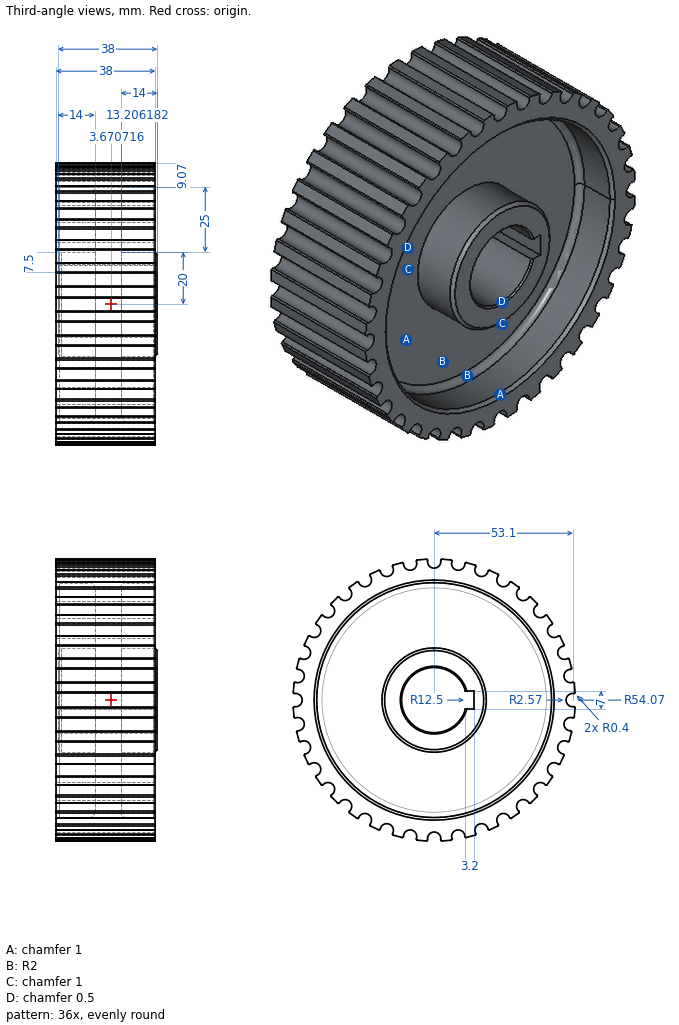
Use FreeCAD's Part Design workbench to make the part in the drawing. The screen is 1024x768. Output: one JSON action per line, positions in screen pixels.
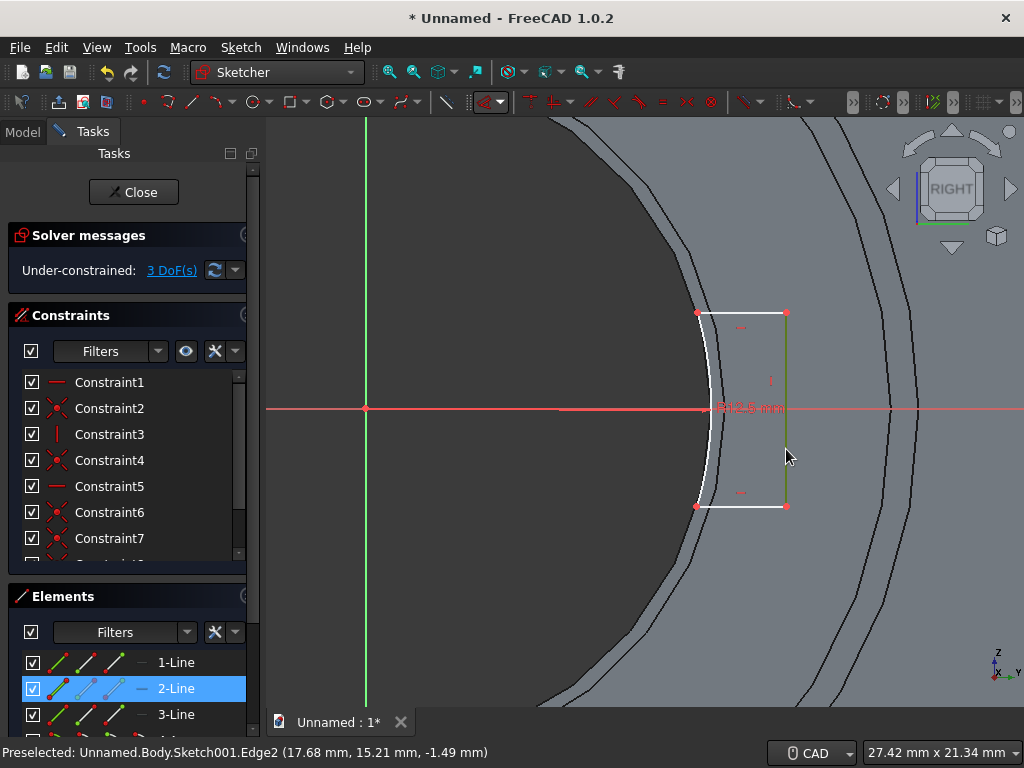
{"action": "key", "text": "i"}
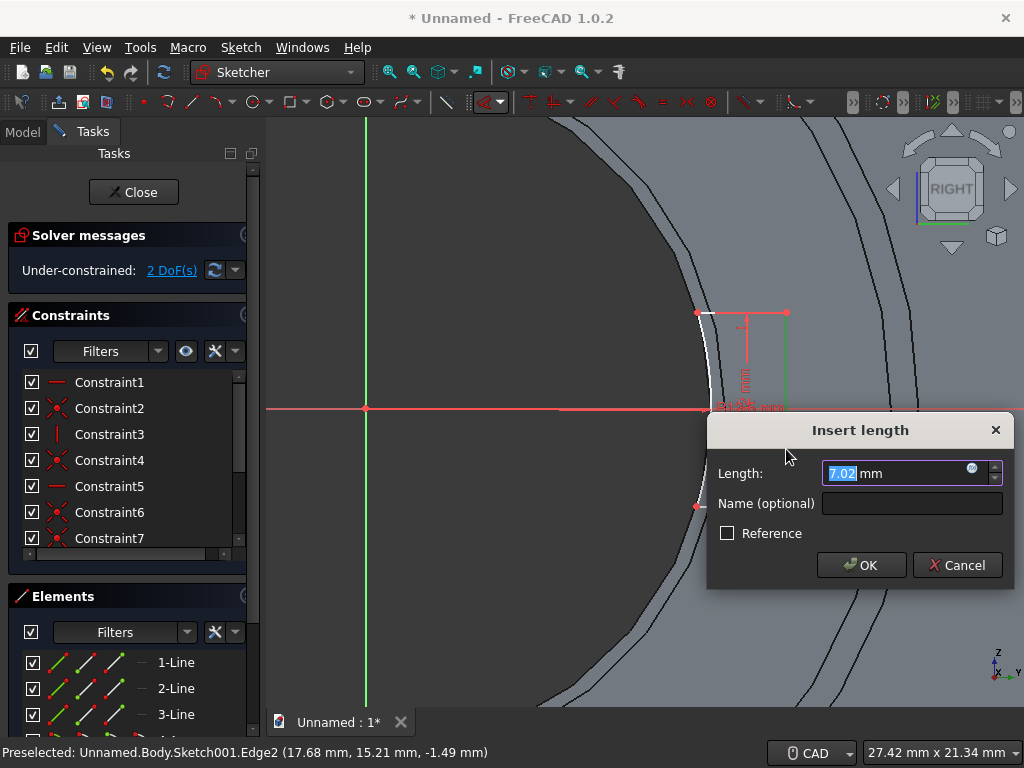
{"action": "type", "text": "7"}
{"action": "key", "text": "Return"}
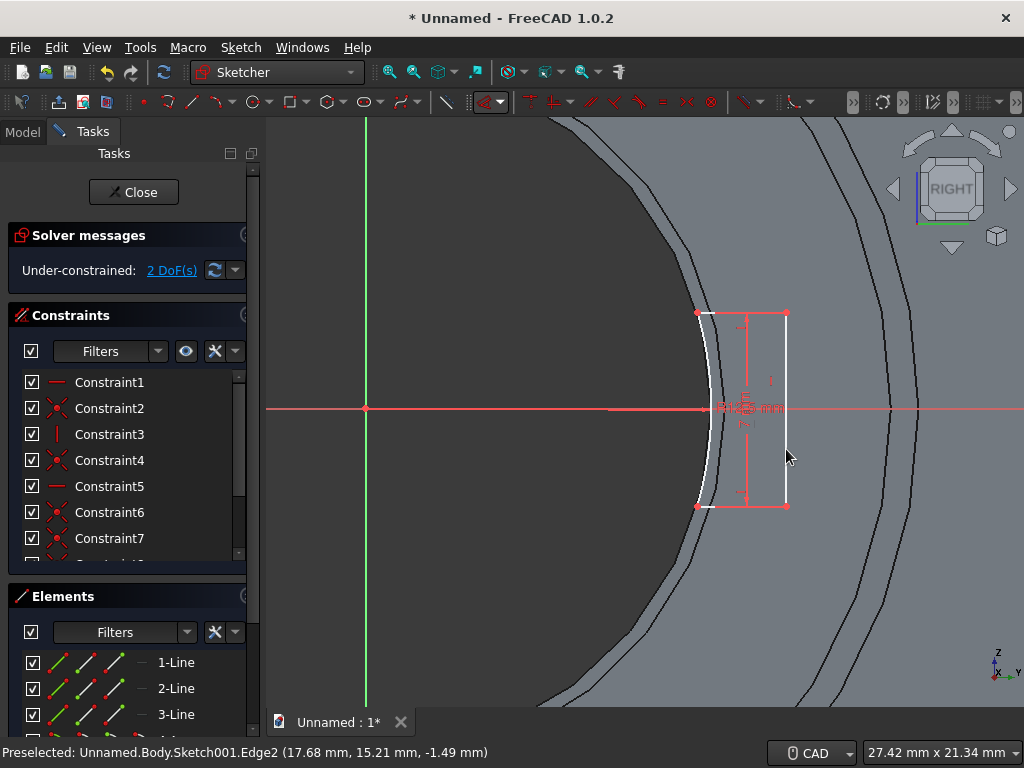
{"action": "left_click", "coordinate": [724, 507]}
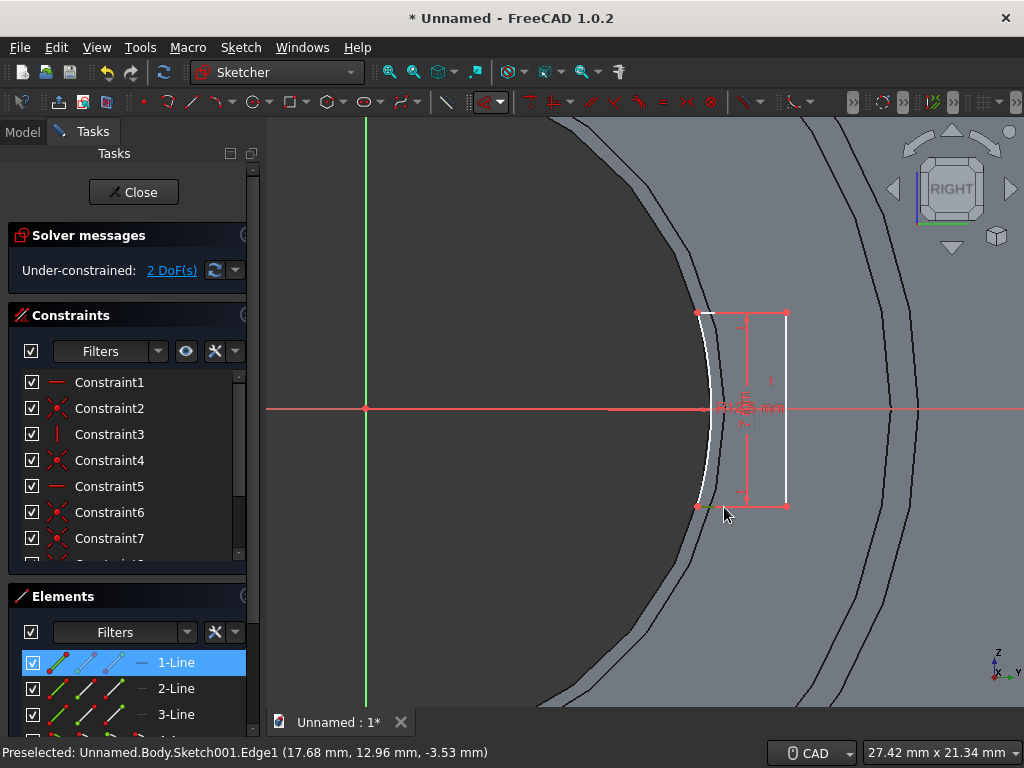
{"action": "left_click", "coordinate": [502, 102]}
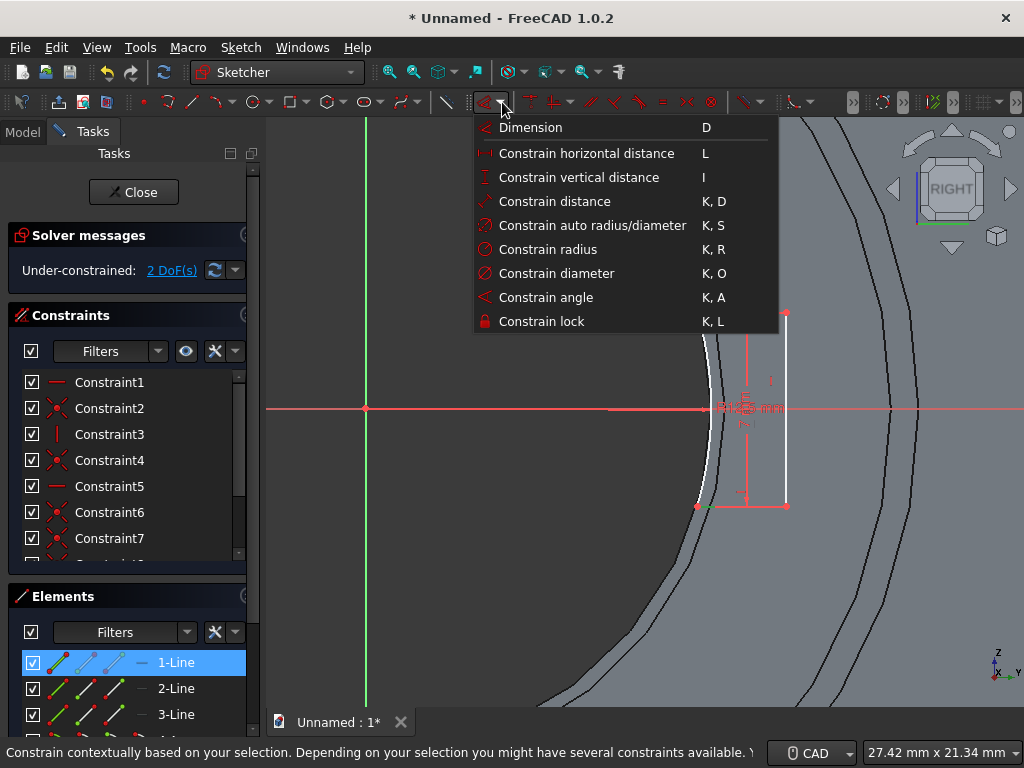
{"action": "left_click", "coordinate": [626, 153]}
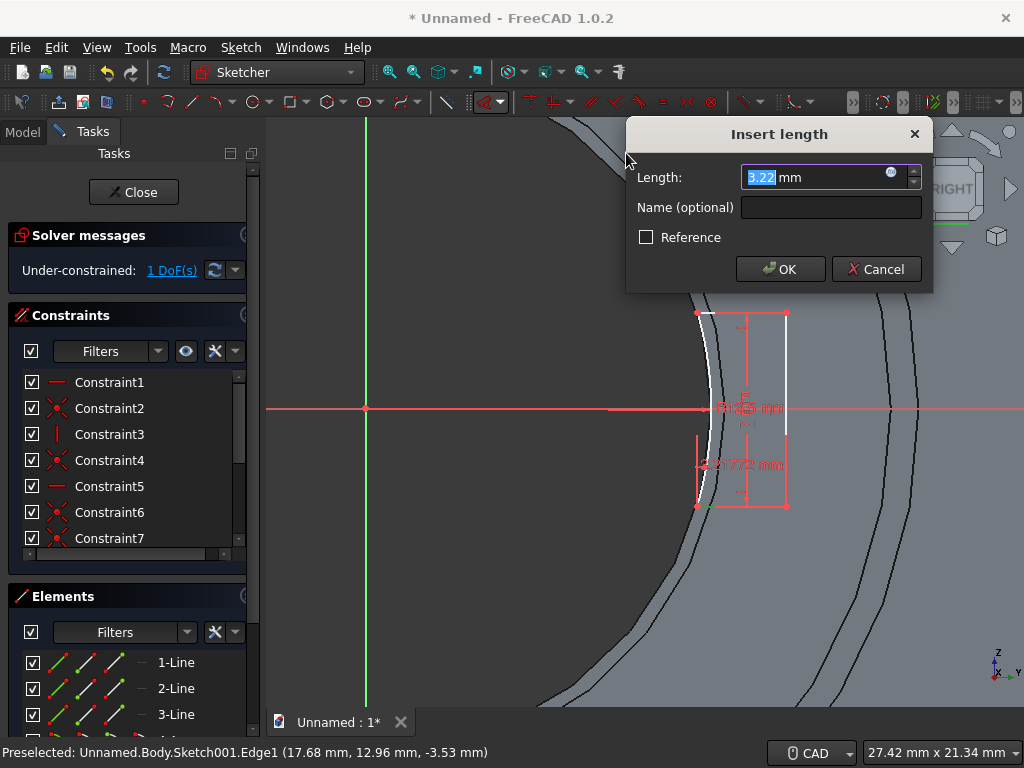
{"action": "type", "text": "3.2"}
{"action": "key", "text": "Return"}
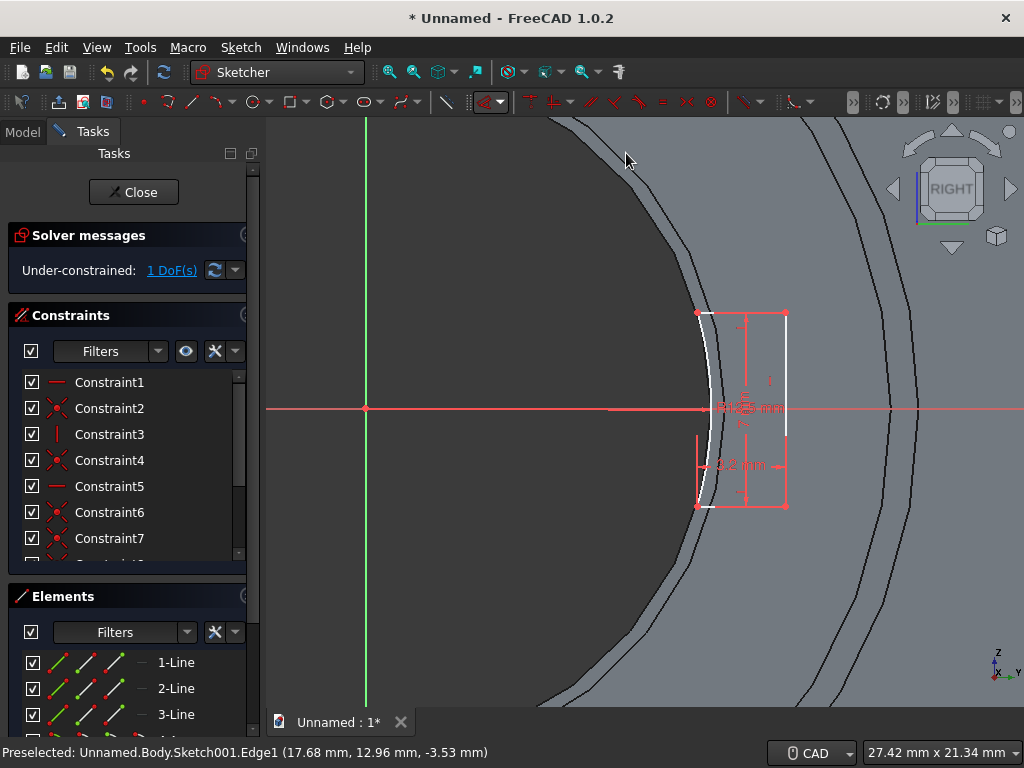
{"action": "left_click", "coordinate": [759, 313]}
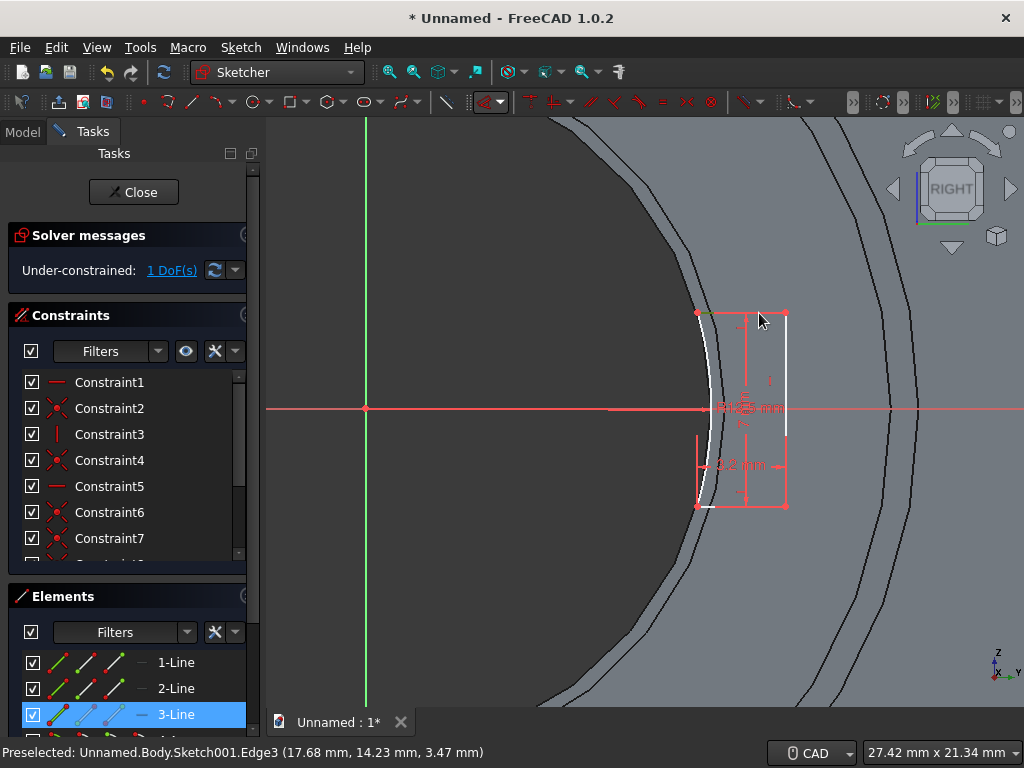
{"action": "key", "text": "l"}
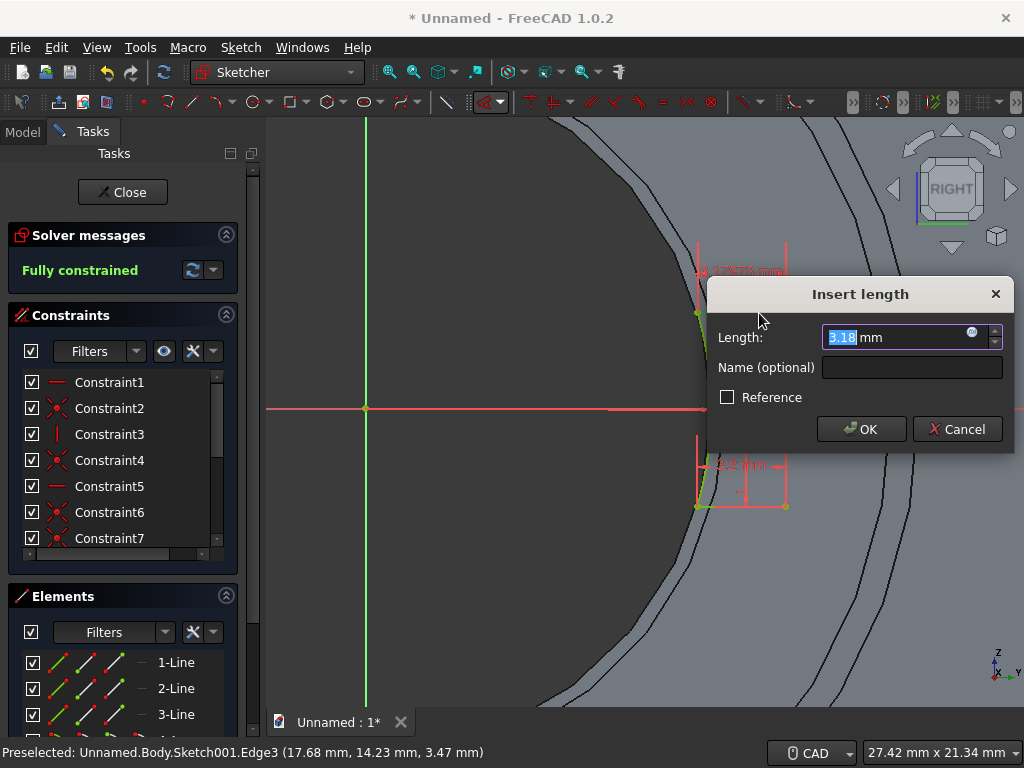
{"action": "type", "text": "3.2"}
{"action": "key", "text": "Return"}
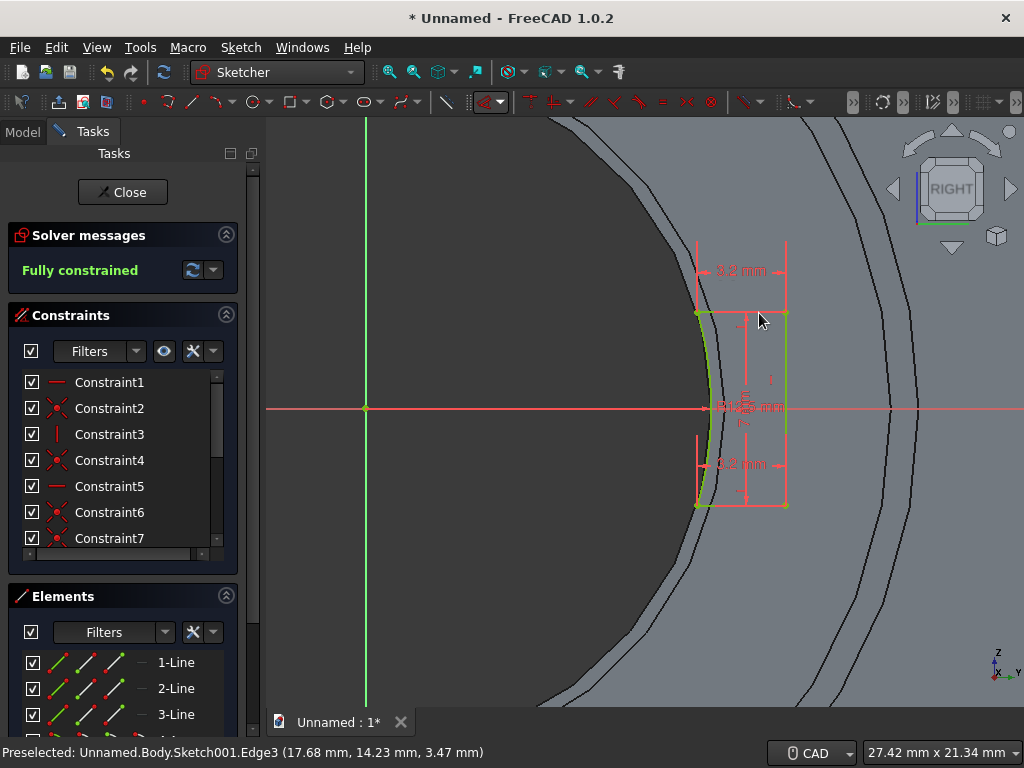
{"action": "left_click", "coordinate": [123, 192]}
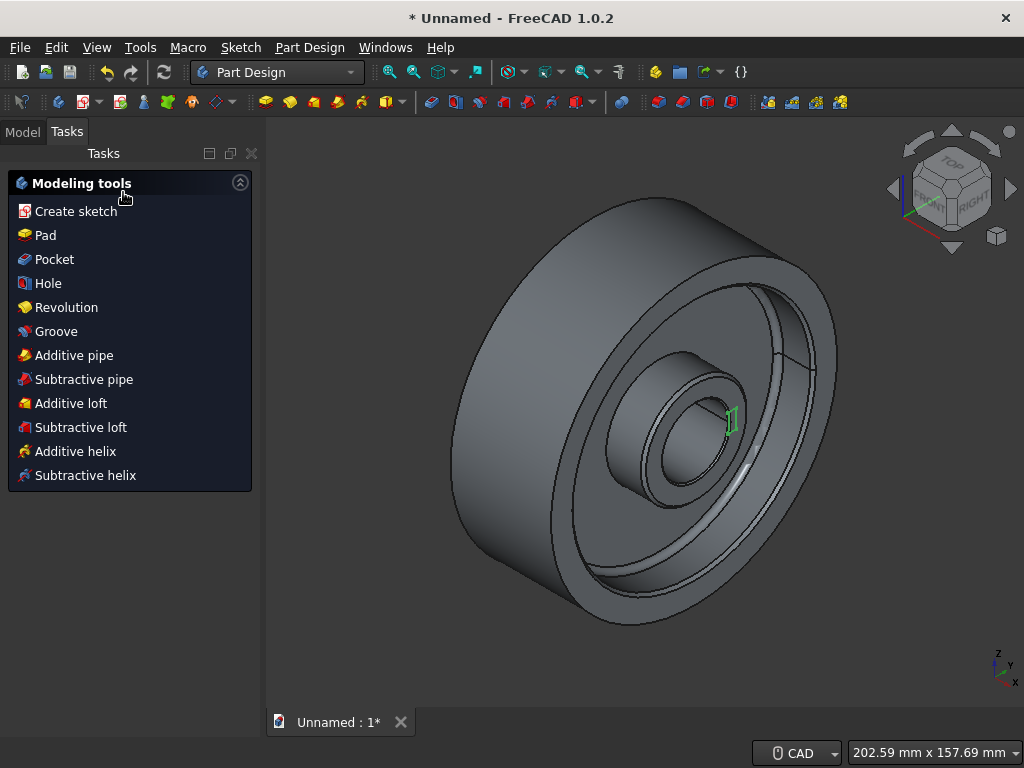
{"action": "left_click", "coordinate": [432, 102]}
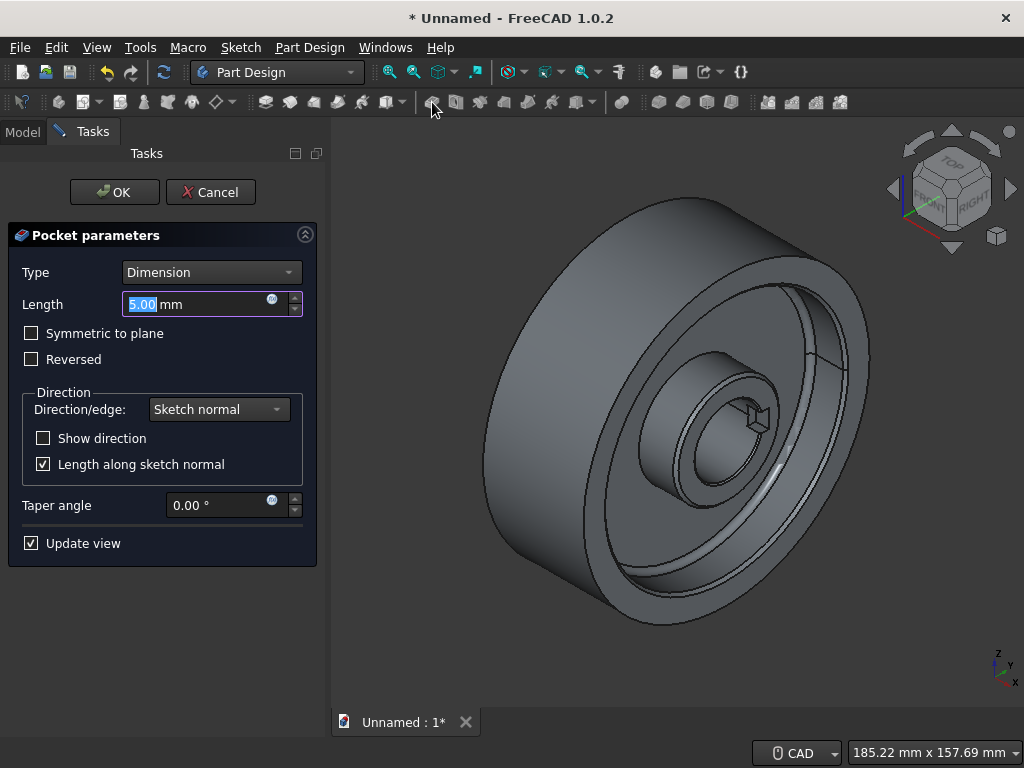
{"action": "left_click", "coordinate": [212, 272]}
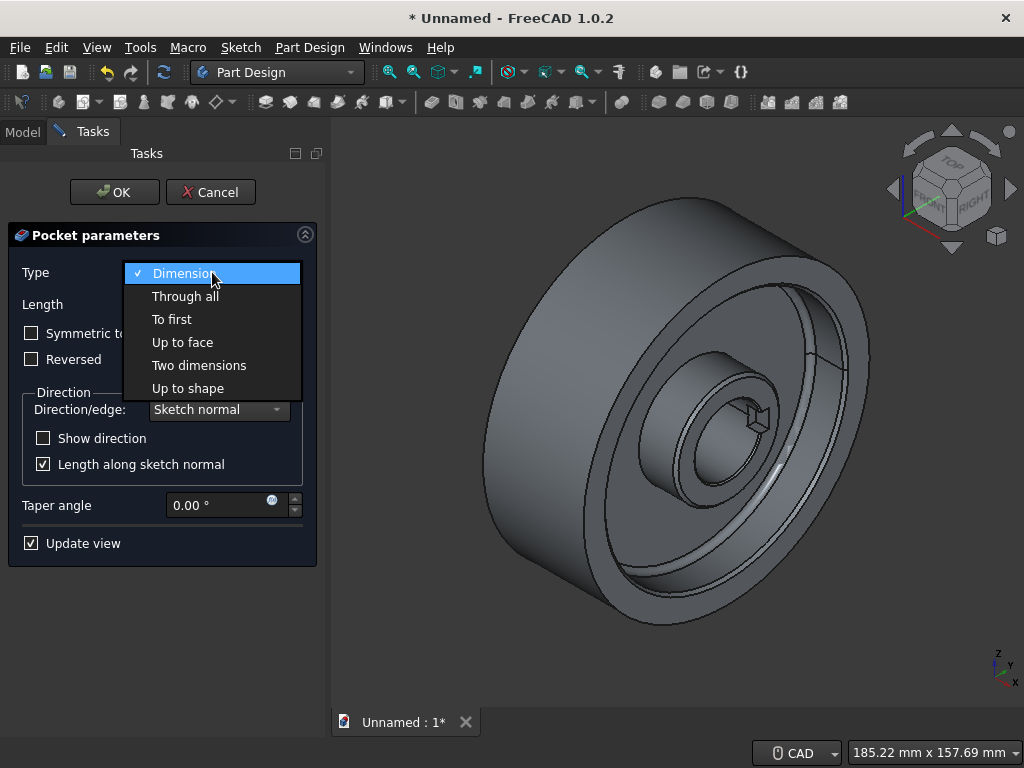
{"action": "left_click", "coordinate": [212, 296]}